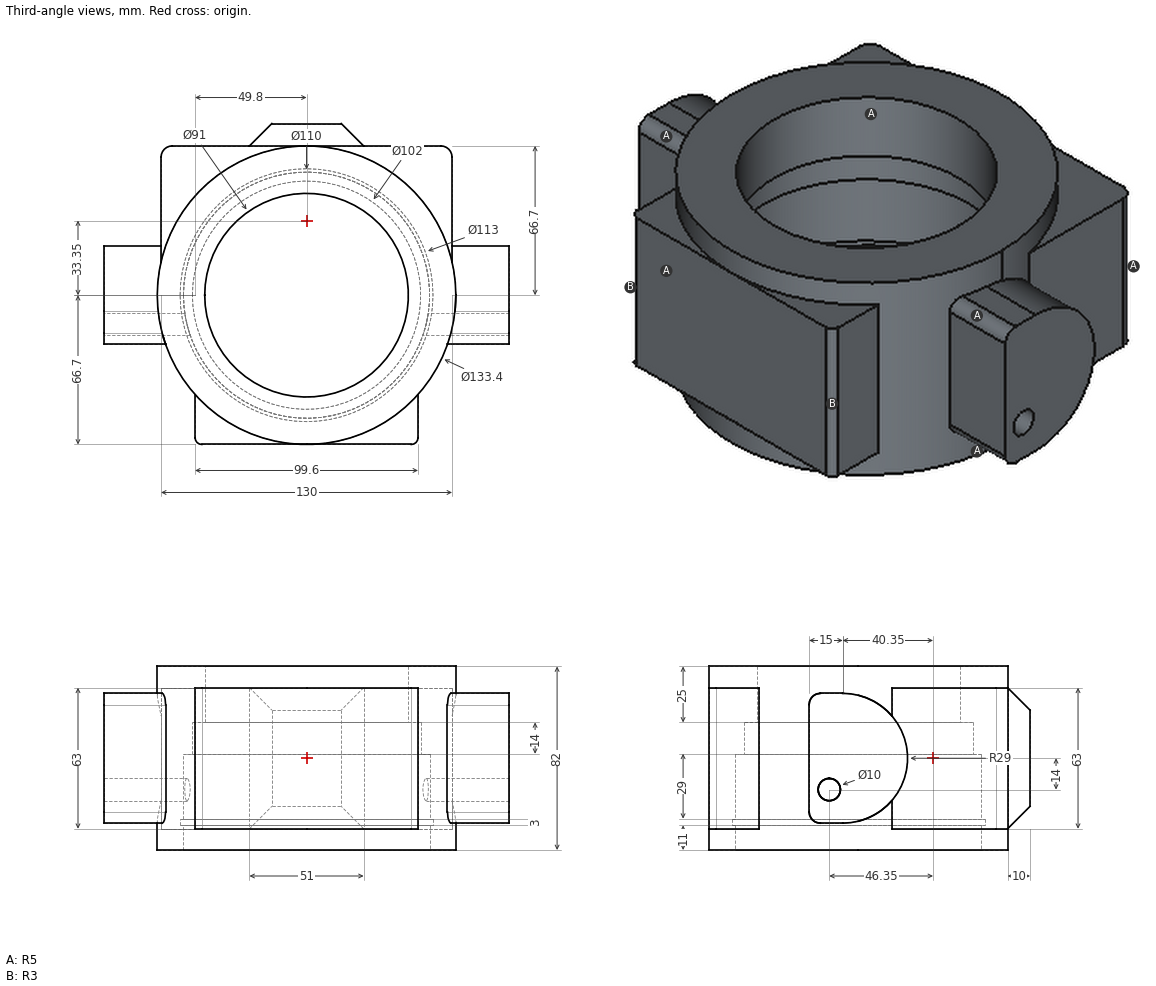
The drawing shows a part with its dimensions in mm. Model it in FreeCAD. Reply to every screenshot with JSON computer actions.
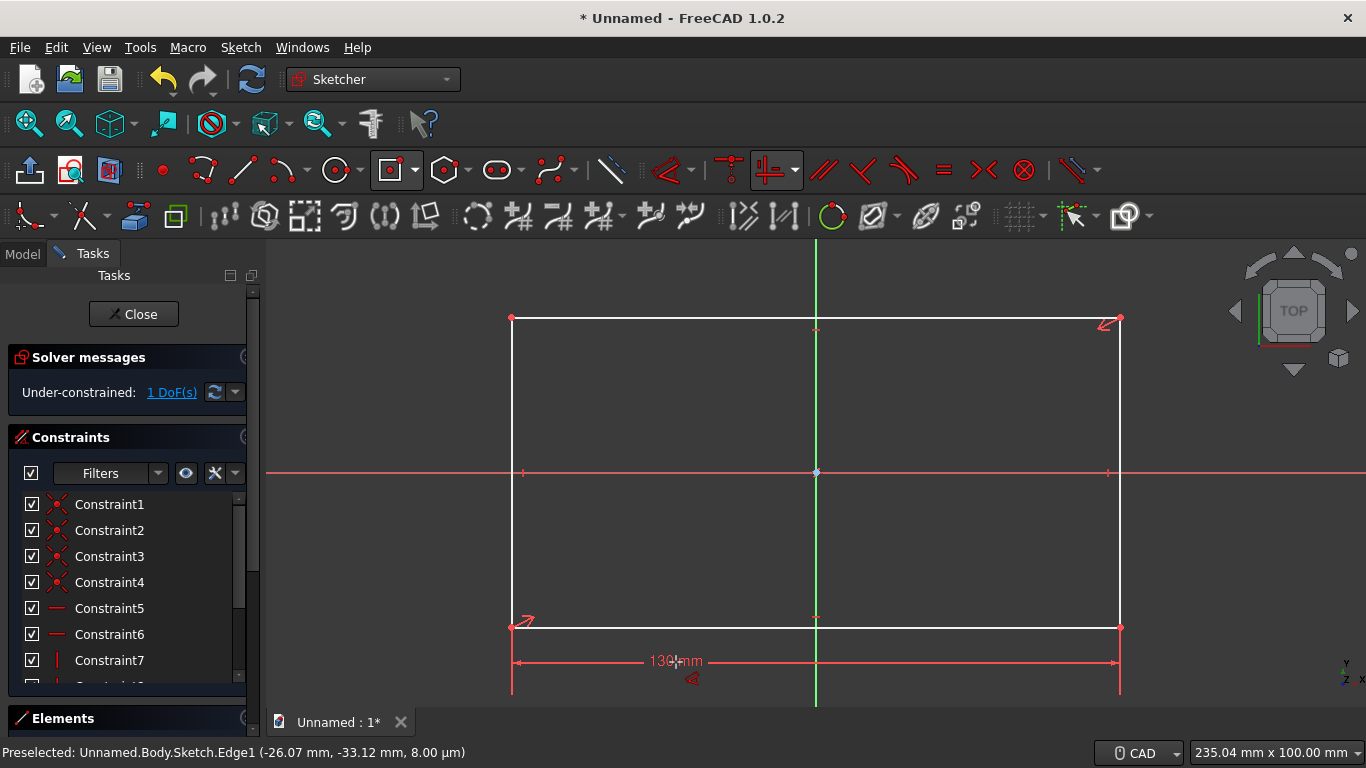
{"action": "left_click", "coordinate": [1120, 535]}
{"action": "left_click", "coordinate": [1154, 402]}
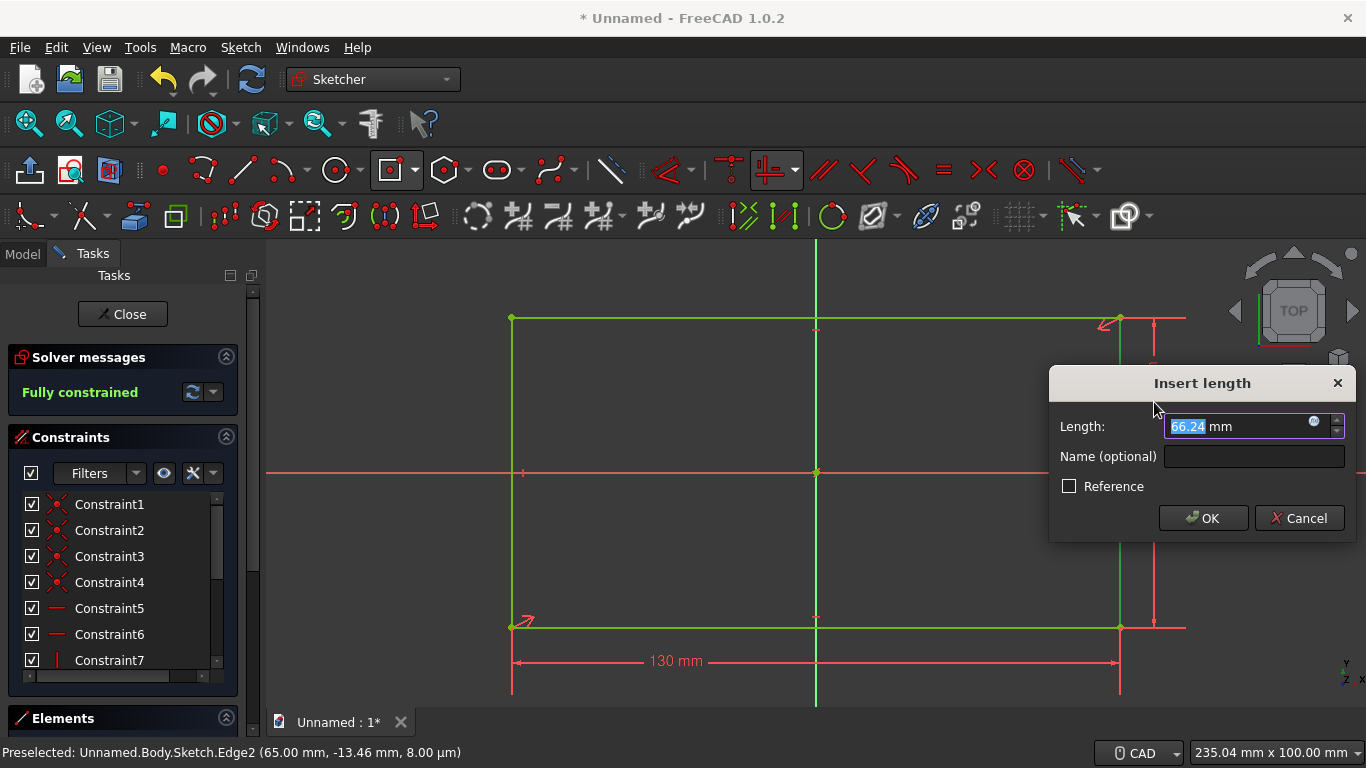
{"action": "type", "text": "66.7"}
{"action": "key", "text": "Return"}
{"action": "key", "text": "Escape"}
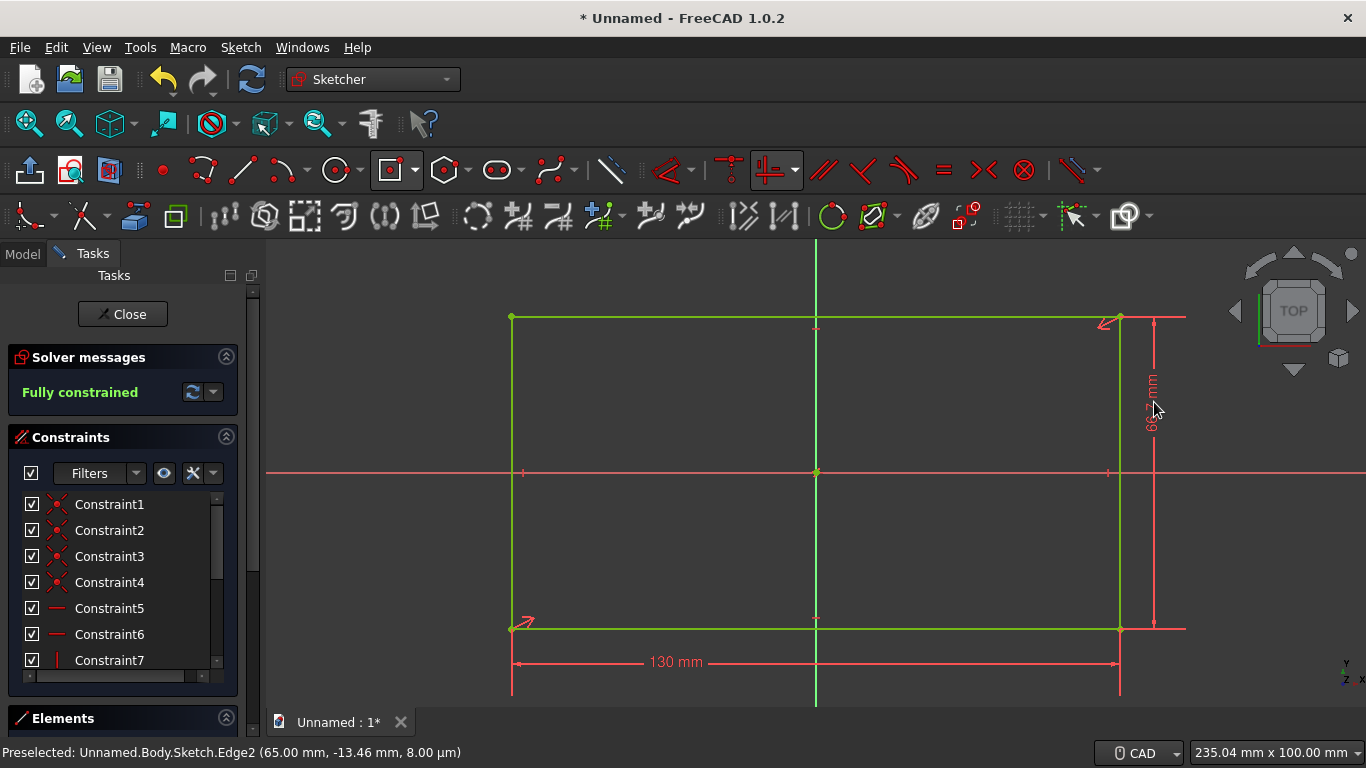
{"action": "left_click", "coordinate": [123, 314]}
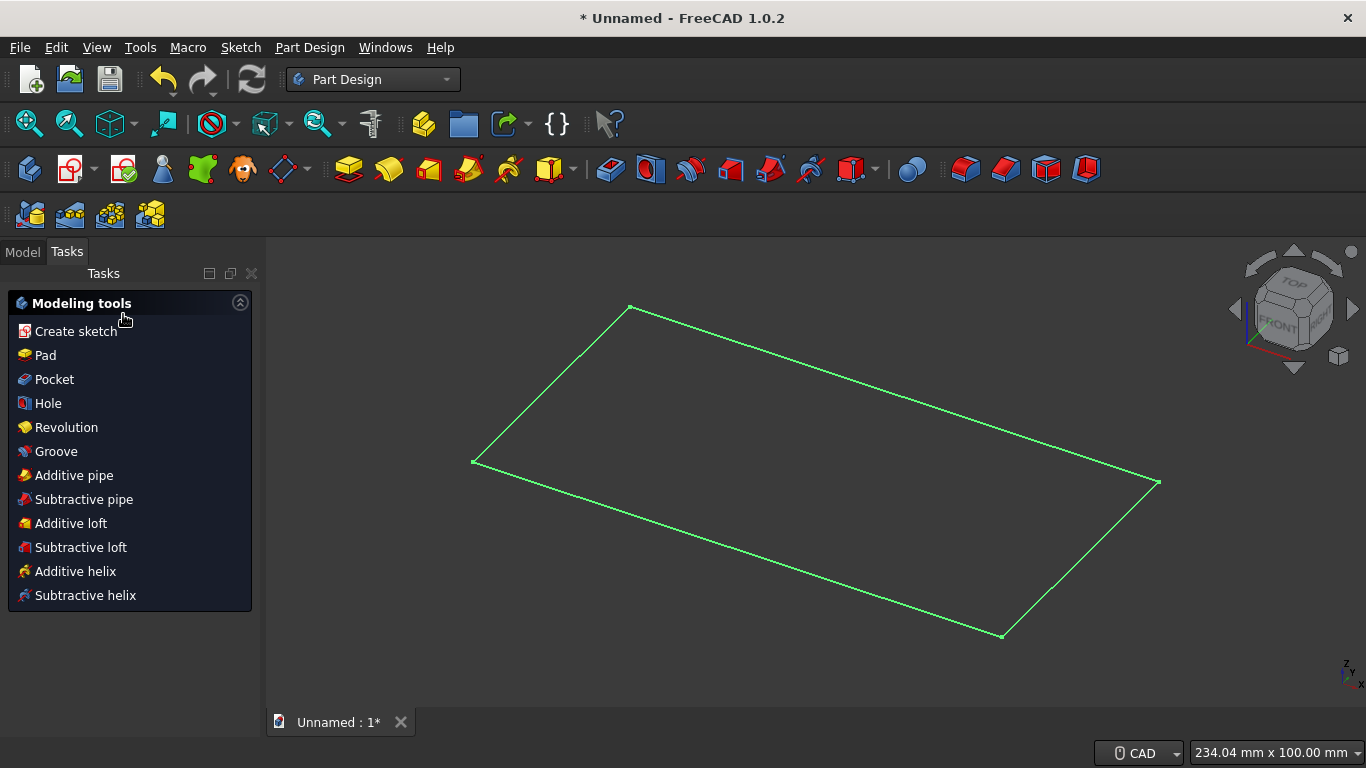
{"action": "left_click", "coordinate": [350, 170]}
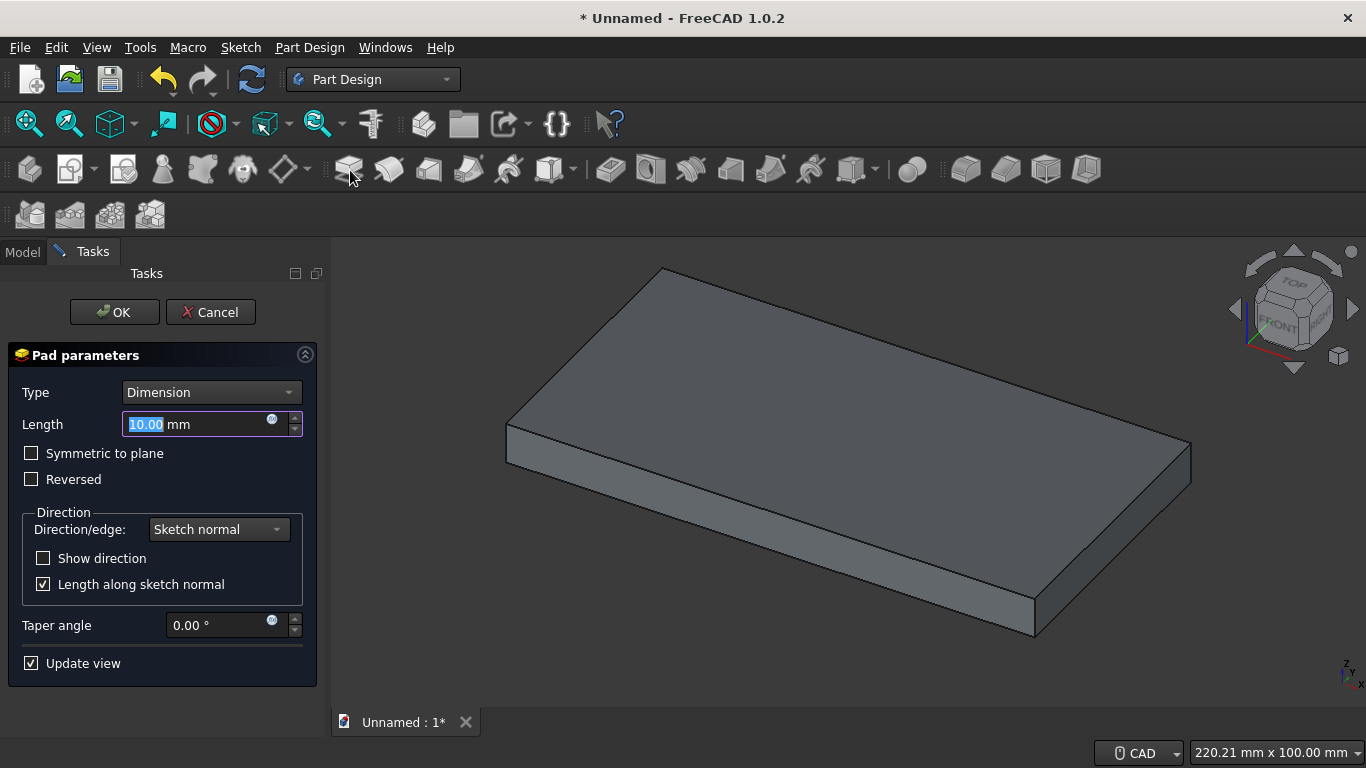
{"action": "type", "text": "63"}
{"action": "key", "text": "Tab"}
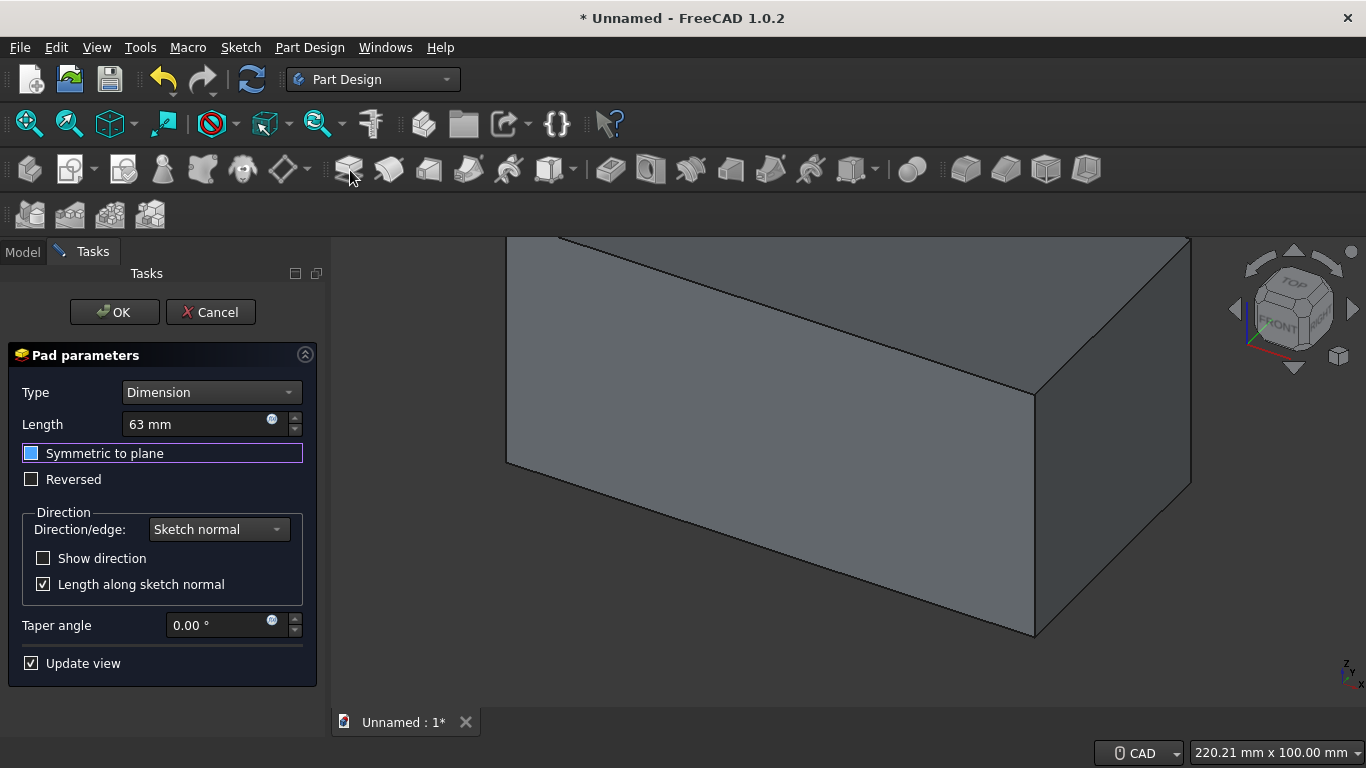
{"action": "left_click", "coordinate": [30, 453]}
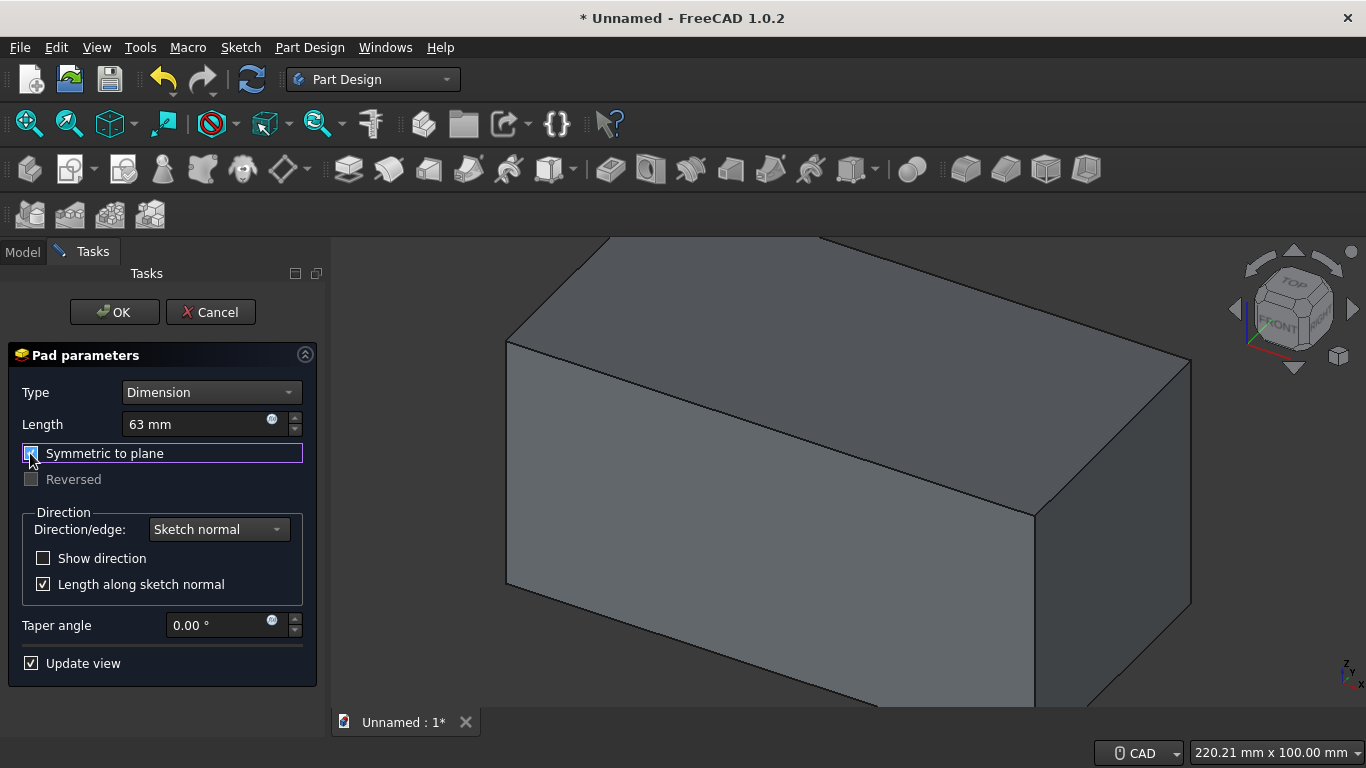
{"action": "left_click", "coordinate": [115, 312]}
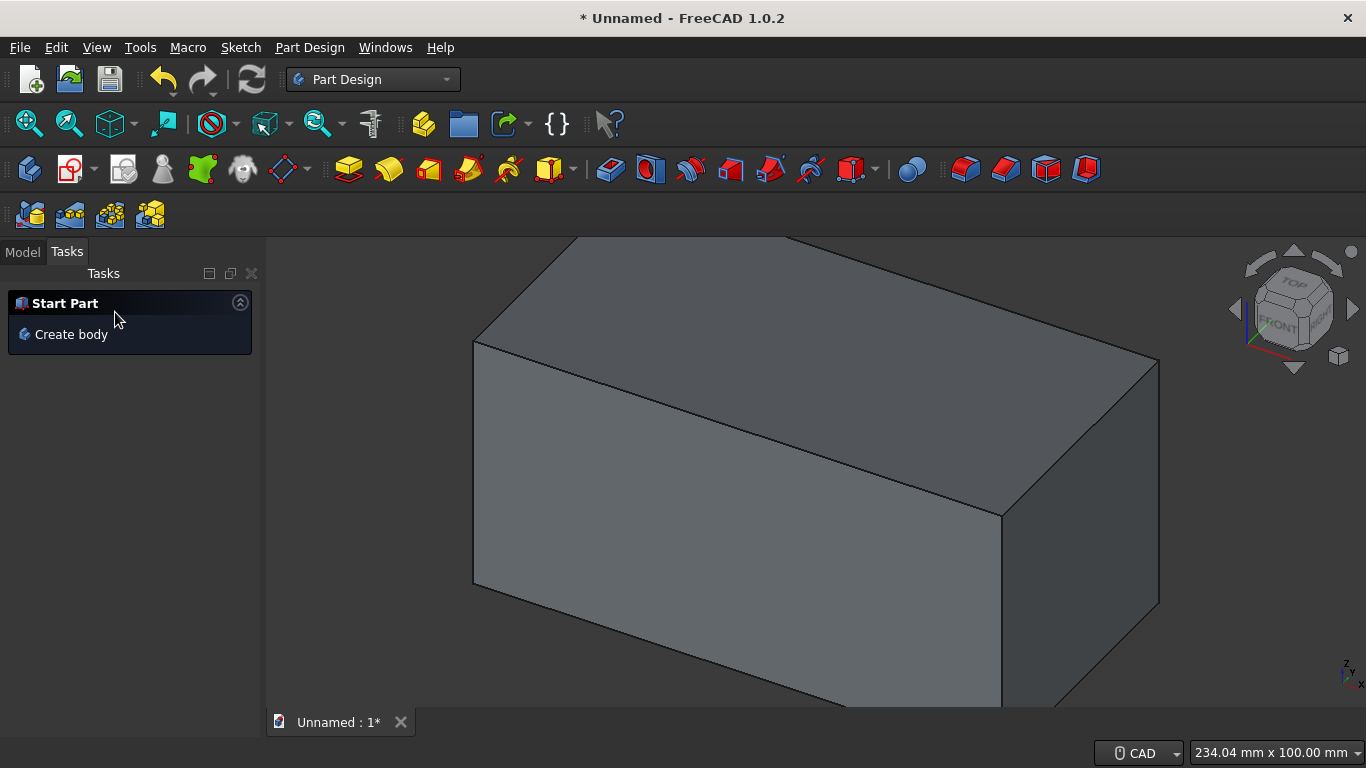
{"action": "key", "text": "v f"}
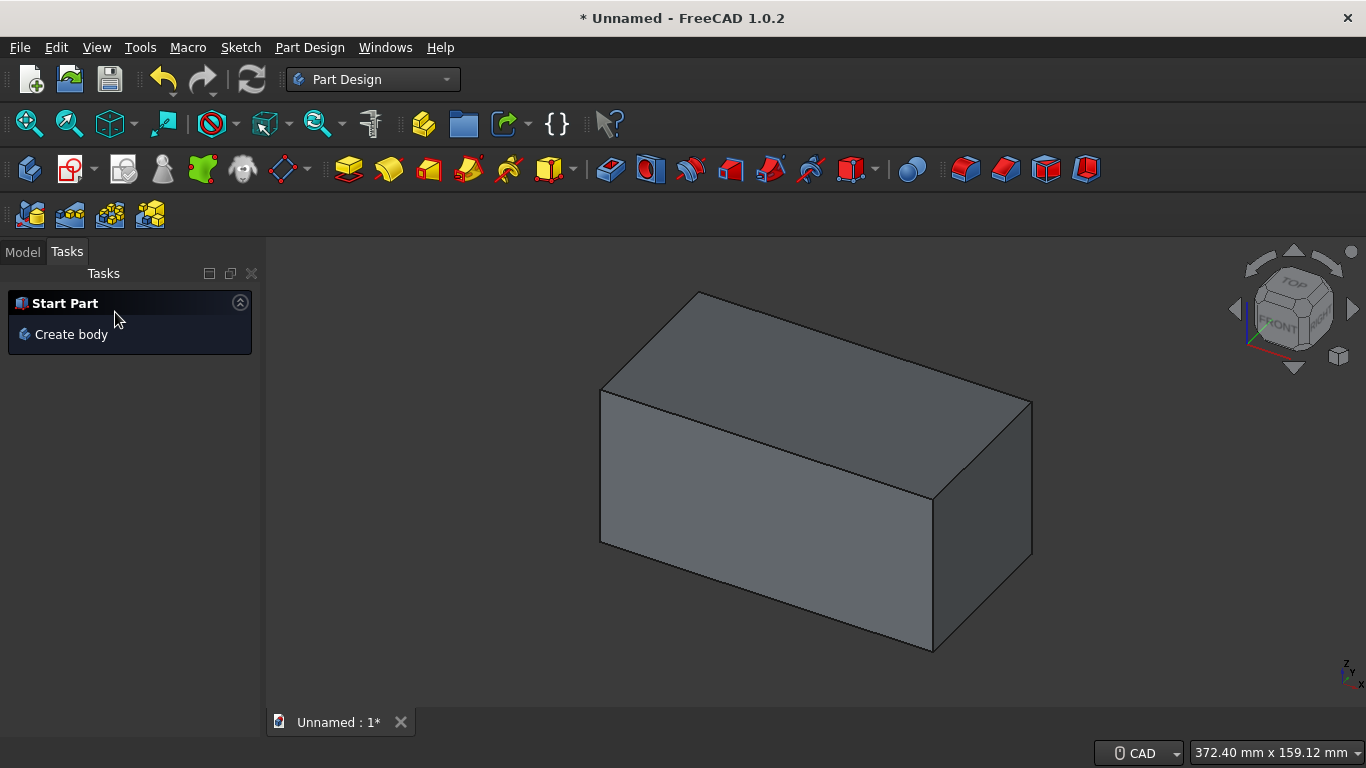
{"action": "key", "text": "4"}